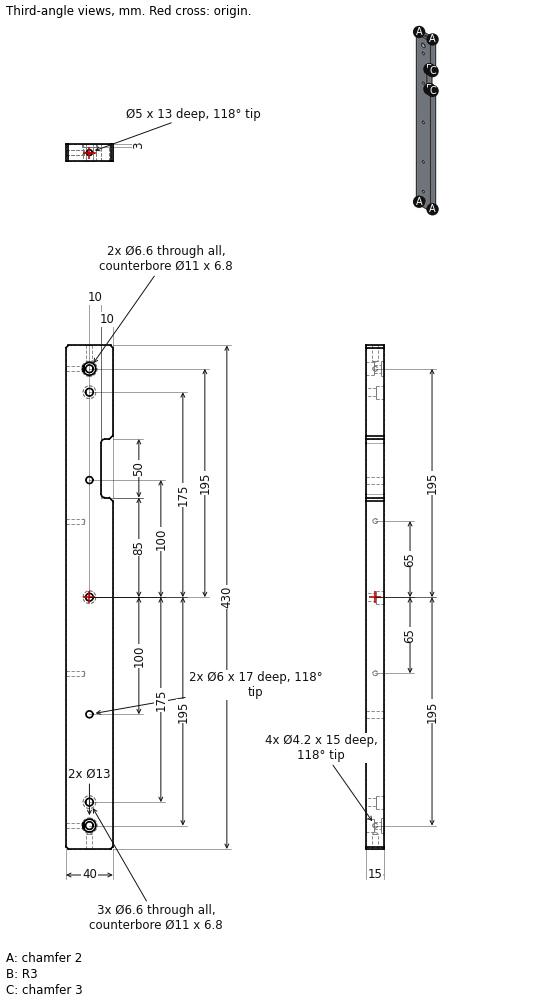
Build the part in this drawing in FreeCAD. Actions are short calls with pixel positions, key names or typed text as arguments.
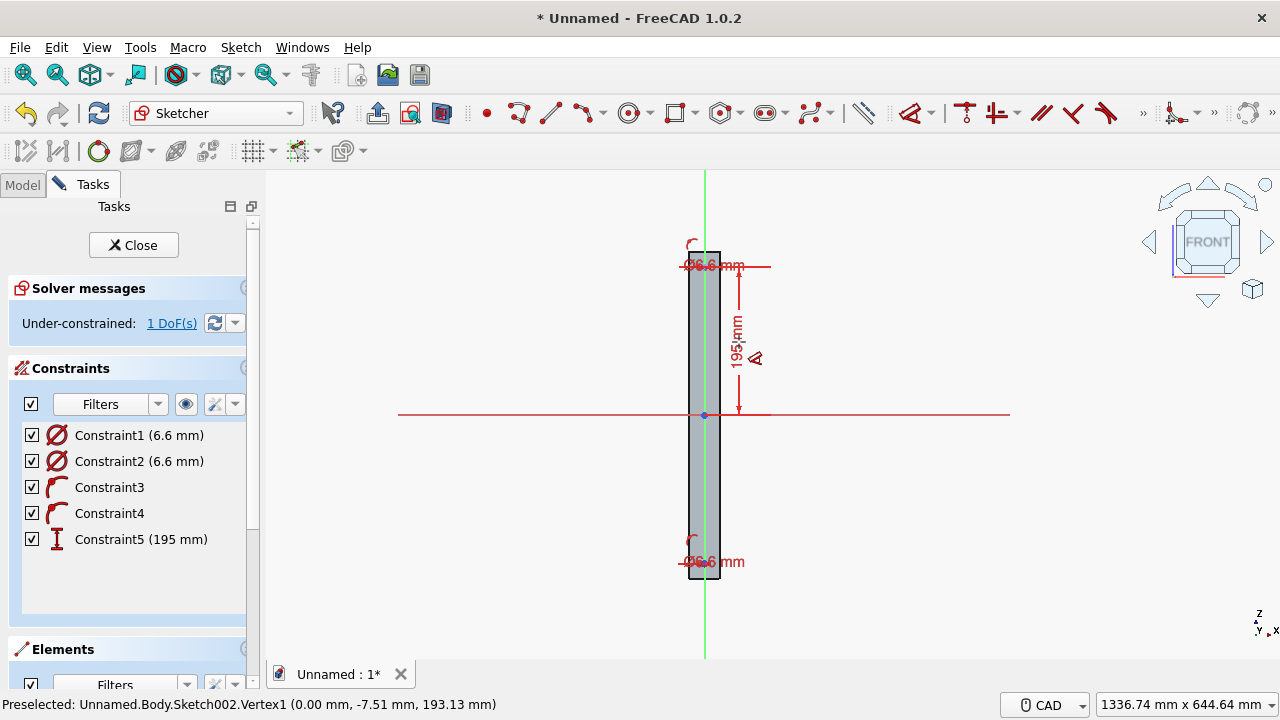
click(705, 564)
click(739, 490)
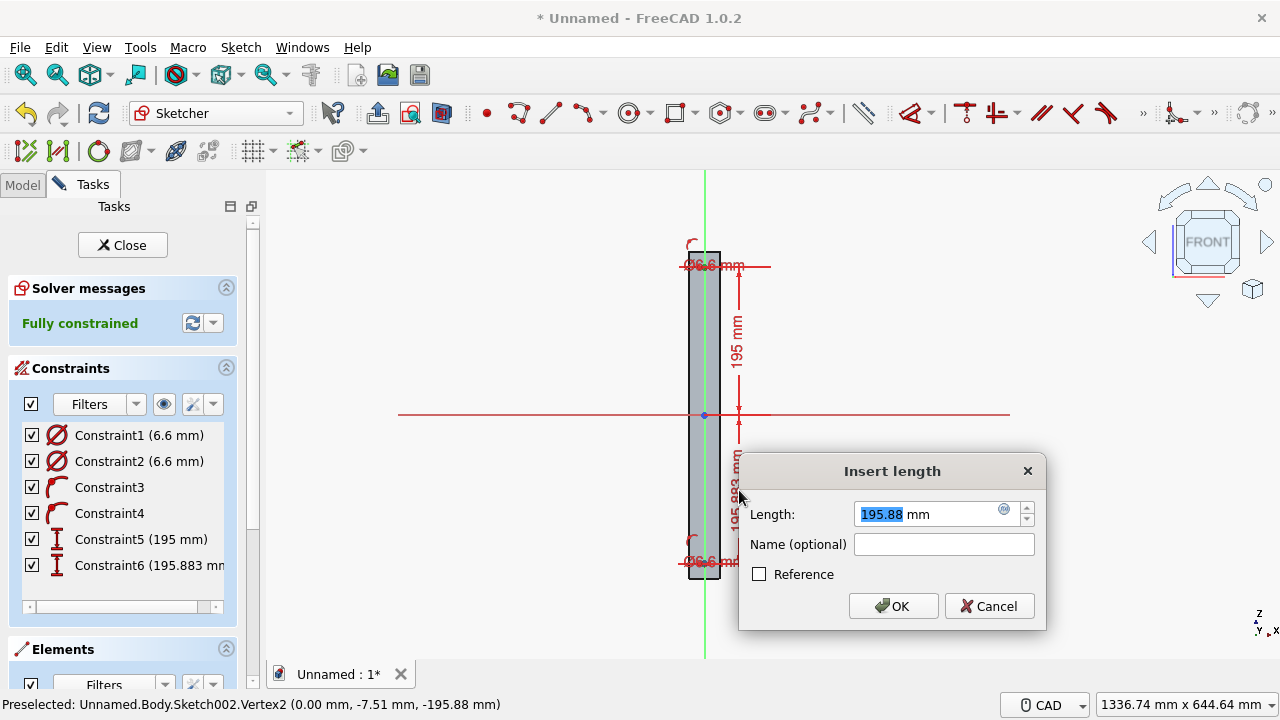
text(195)
key(Return)
key(Escape)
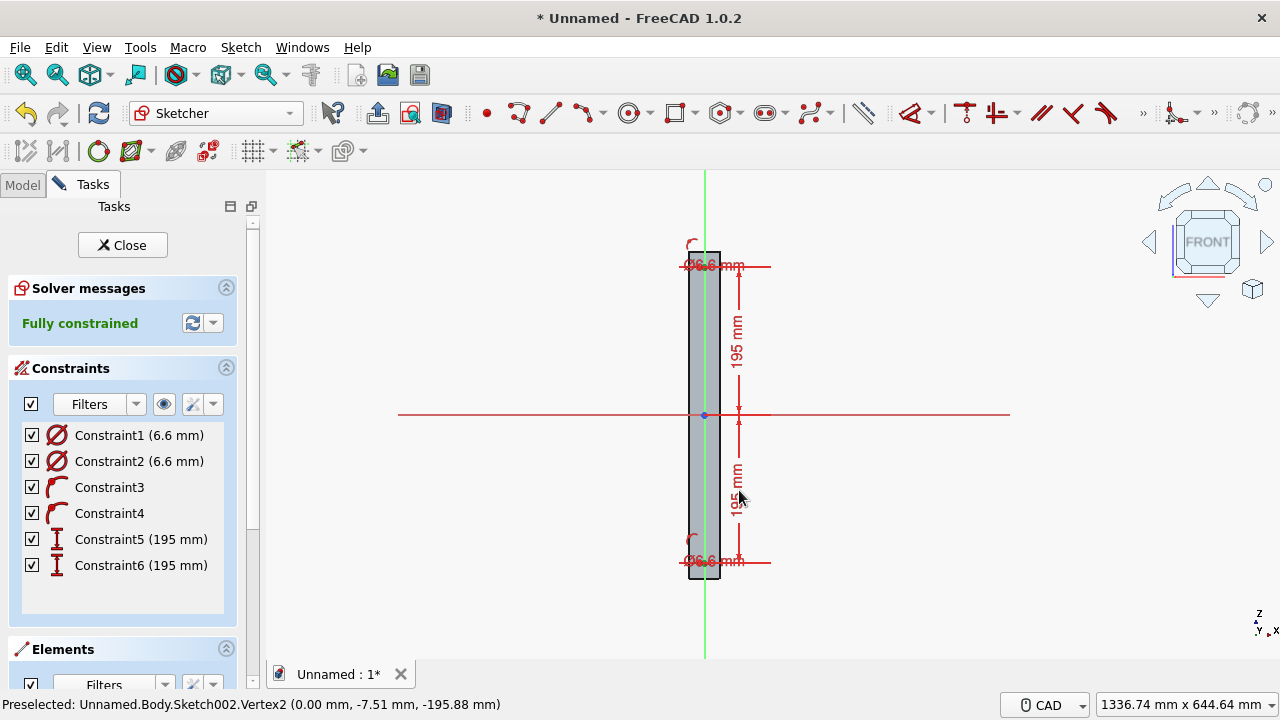
click(123, 245)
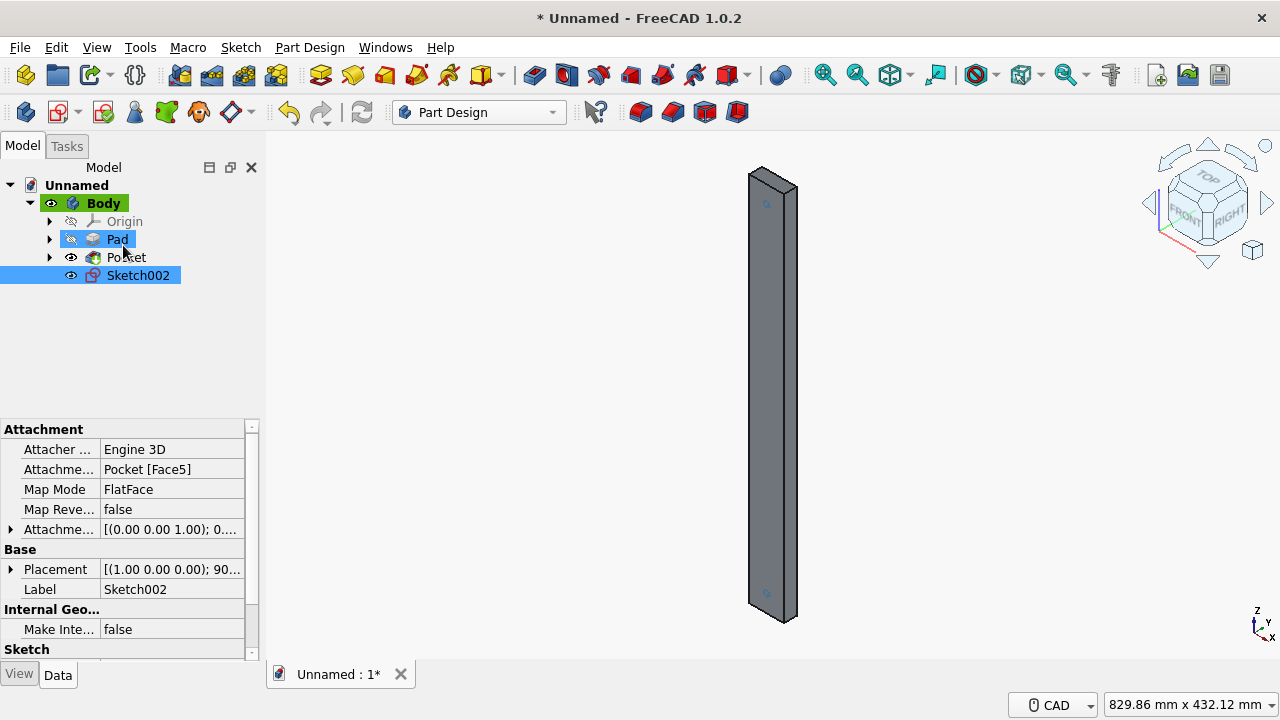
click(568, 76)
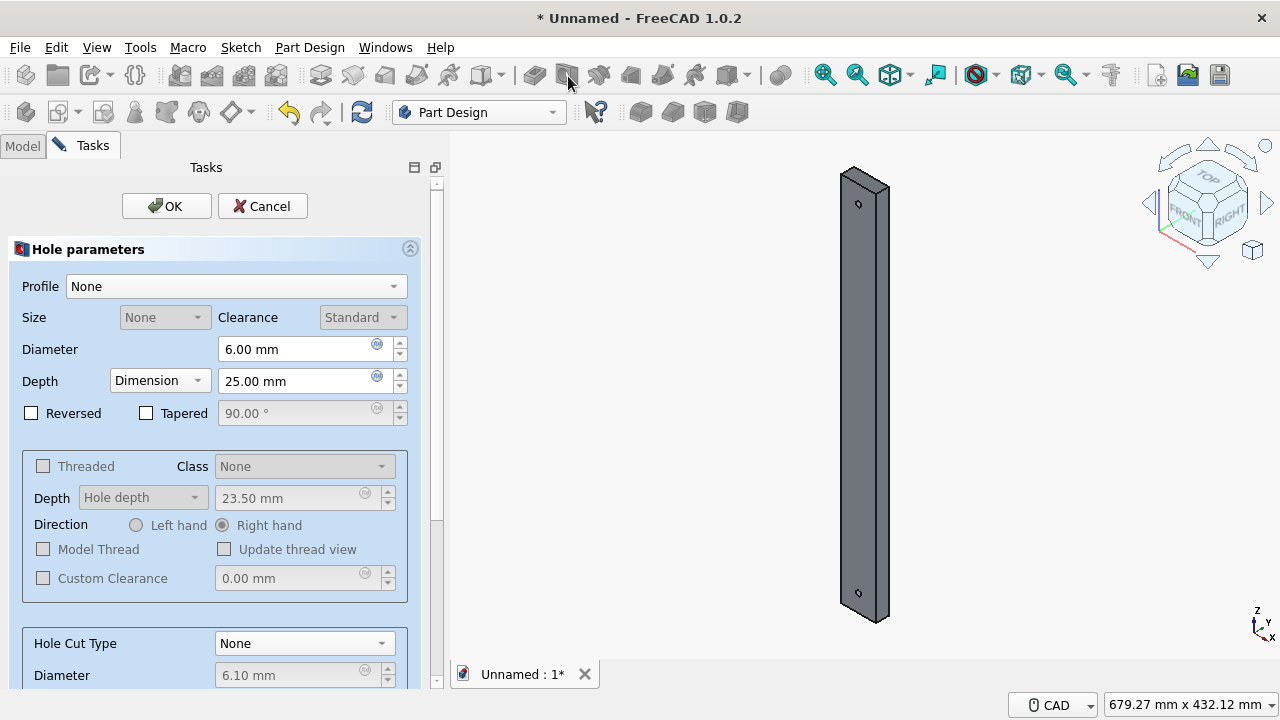
triple_click(305, 349)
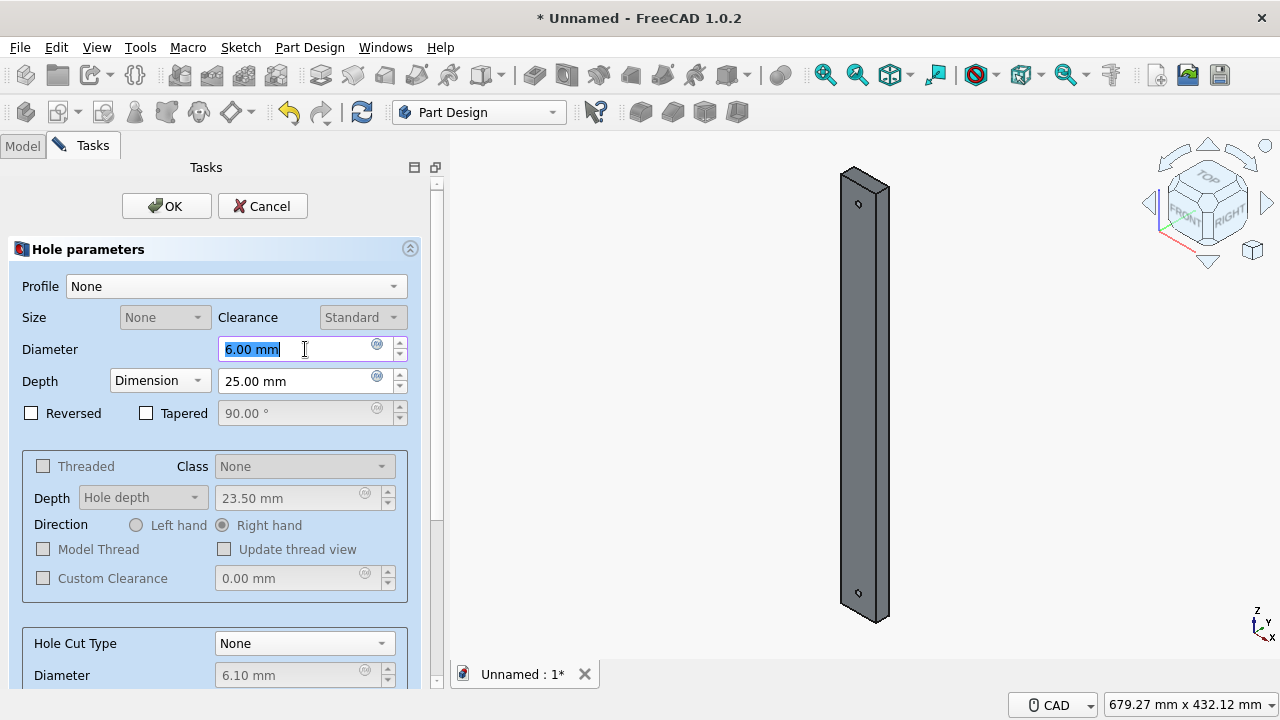
text(6.6)
key(Tab)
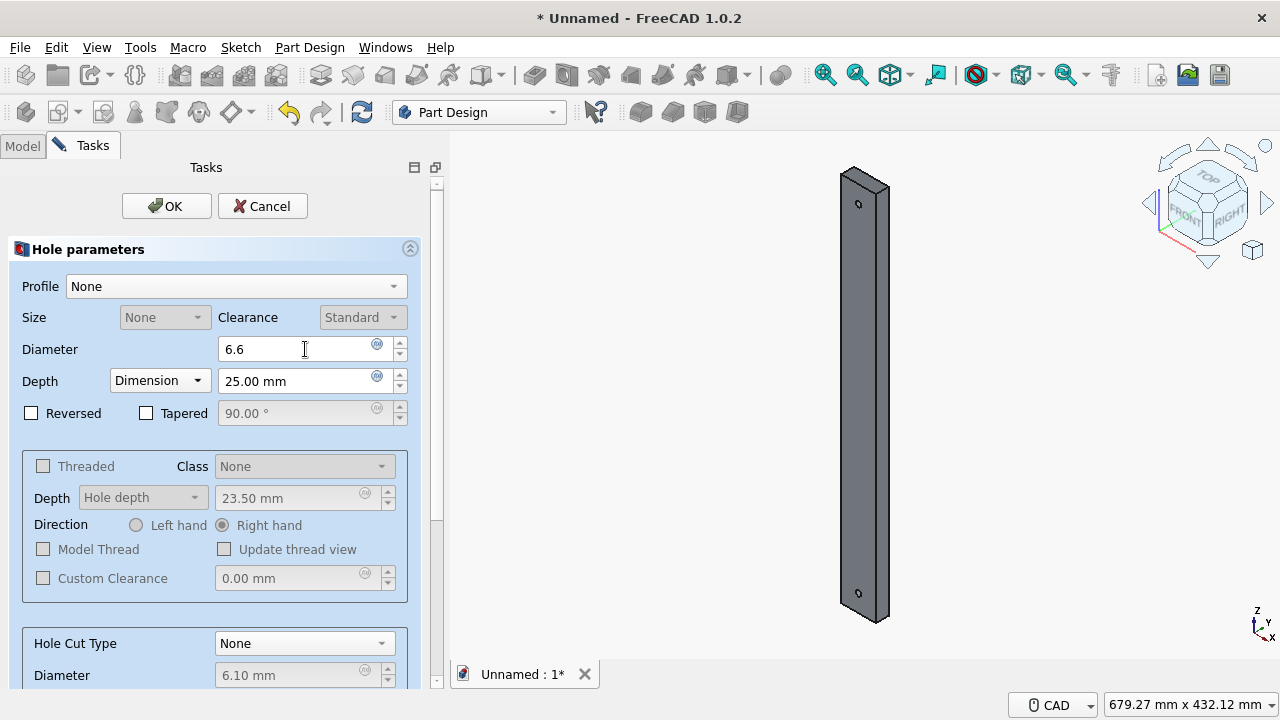
click(161, 380)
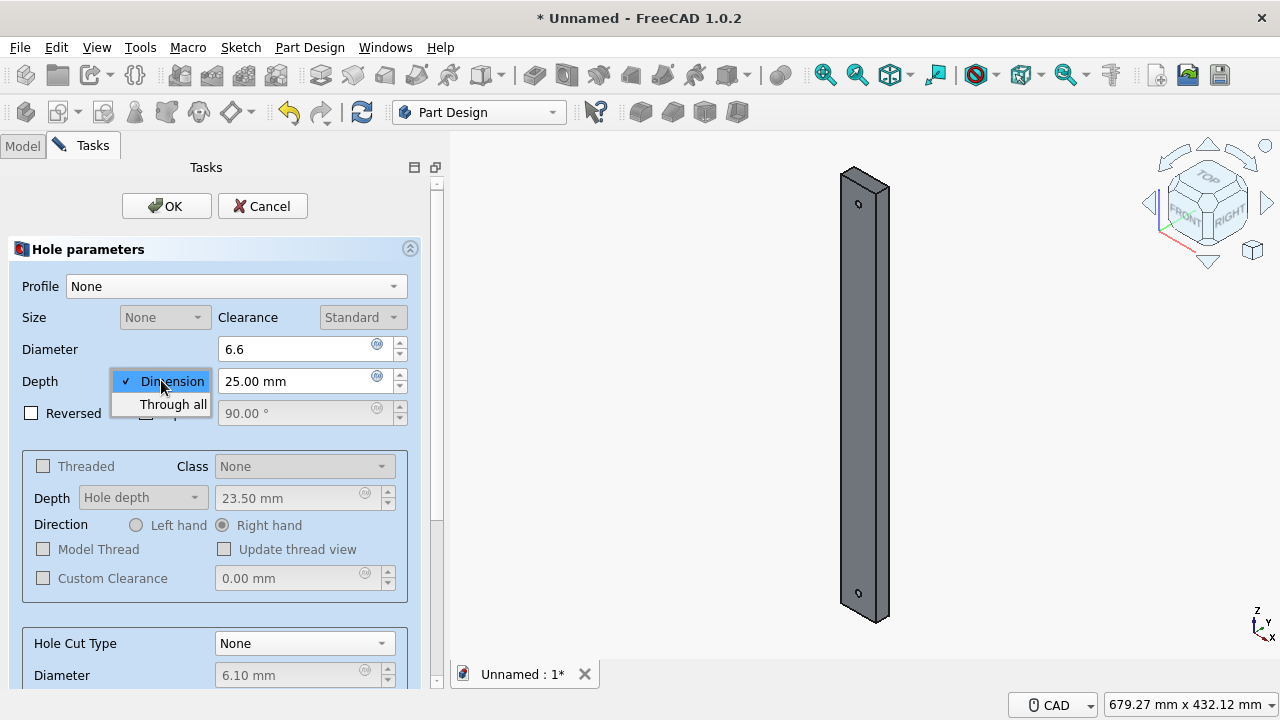
click(160, 404)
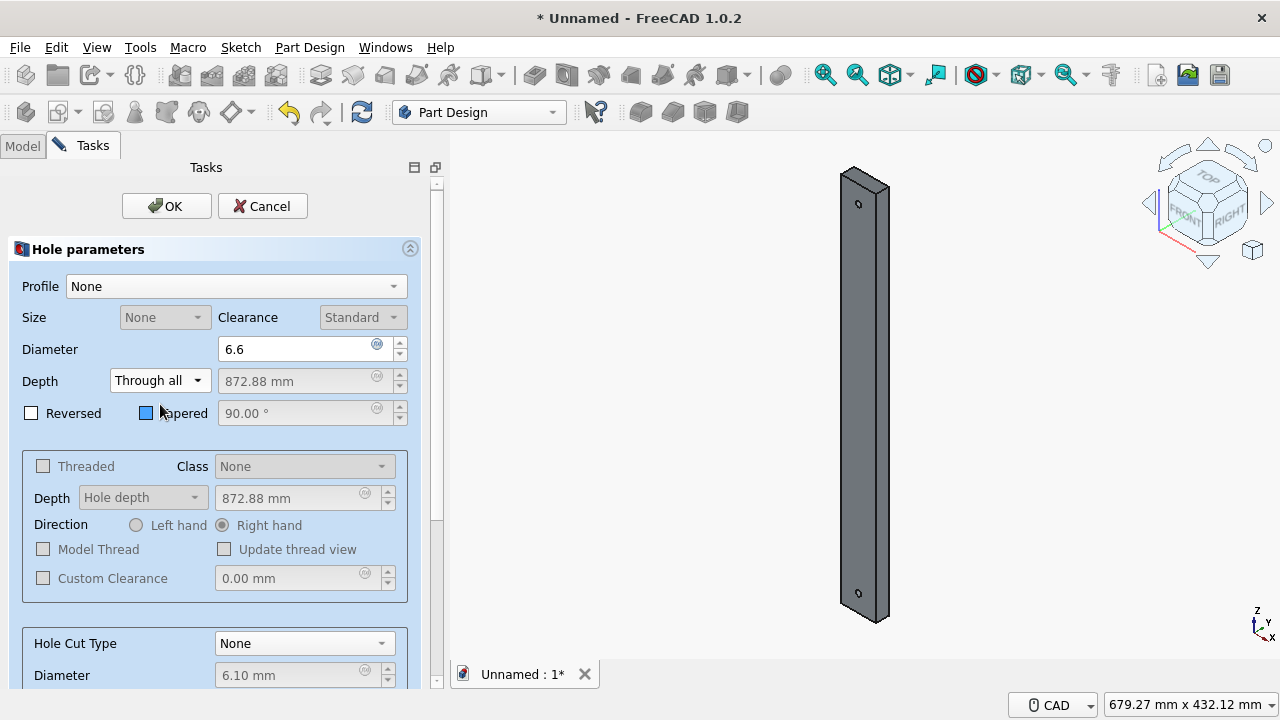
click(306, 644)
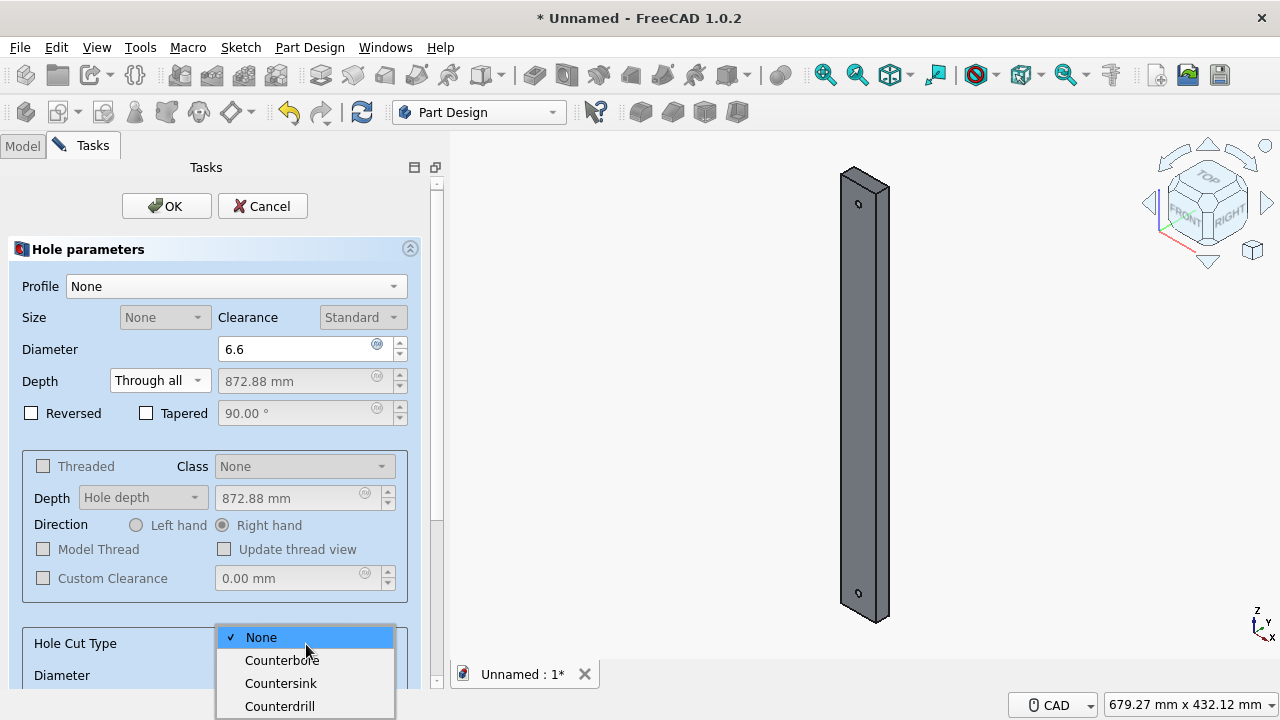
click(304, 660)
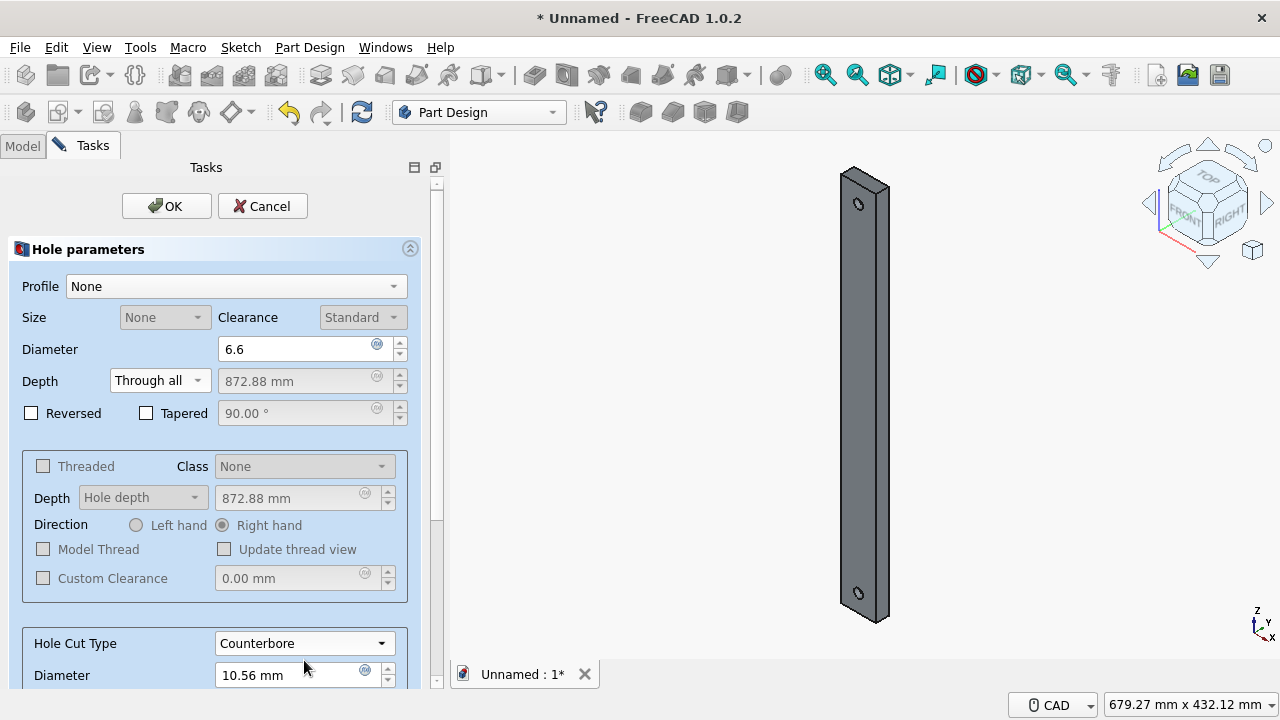
triple_click(298, 675)